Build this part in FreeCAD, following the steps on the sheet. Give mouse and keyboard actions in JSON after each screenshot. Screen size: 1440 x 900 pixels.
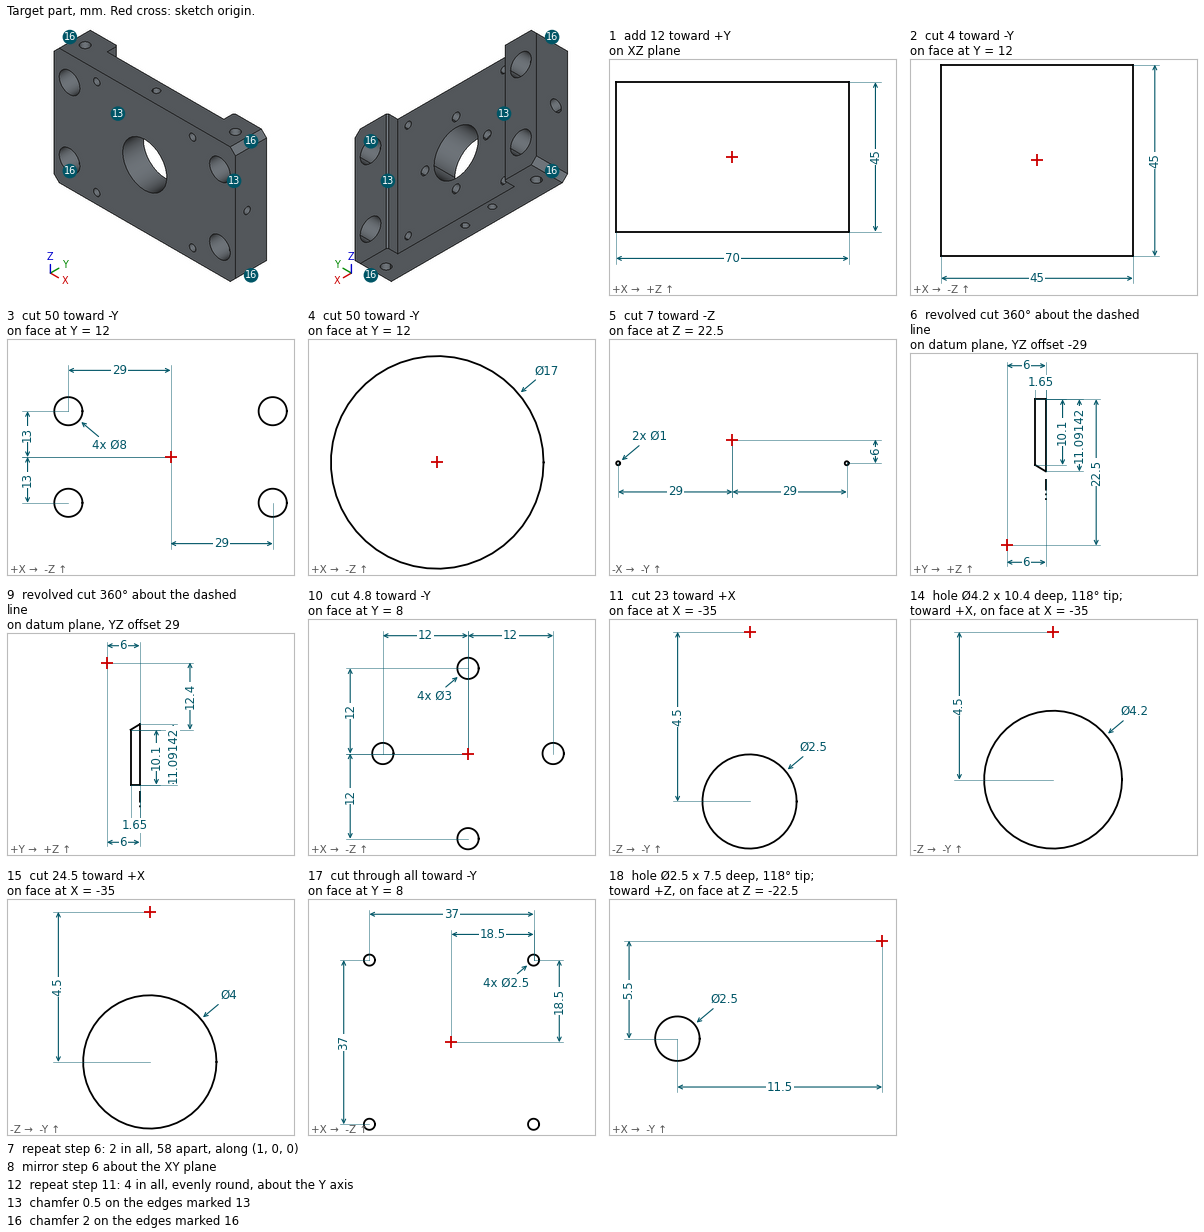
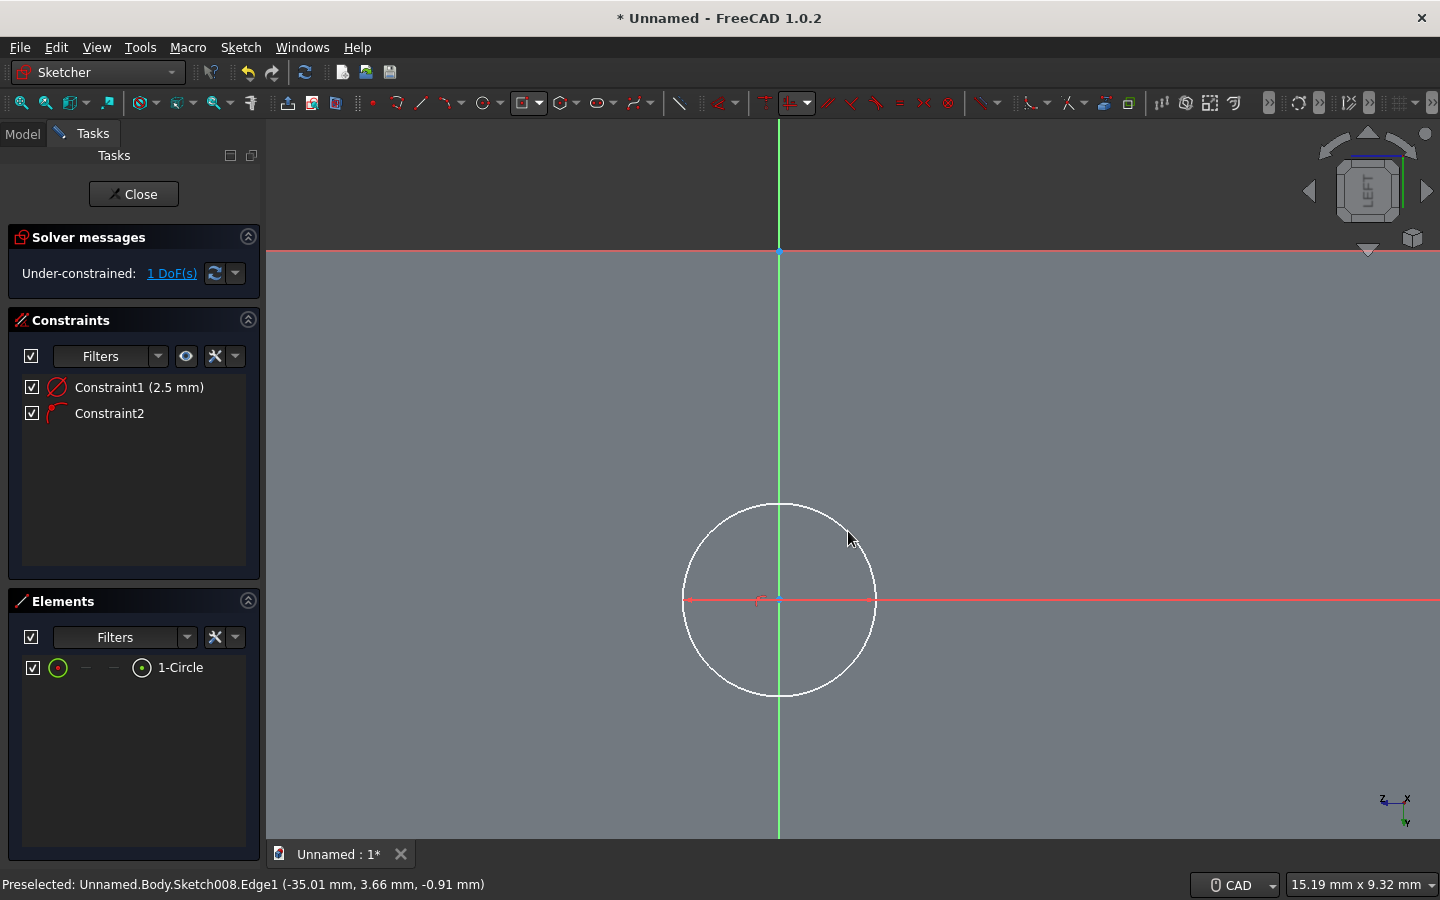
{"action": "left_click", "coordinate": [718, 104]}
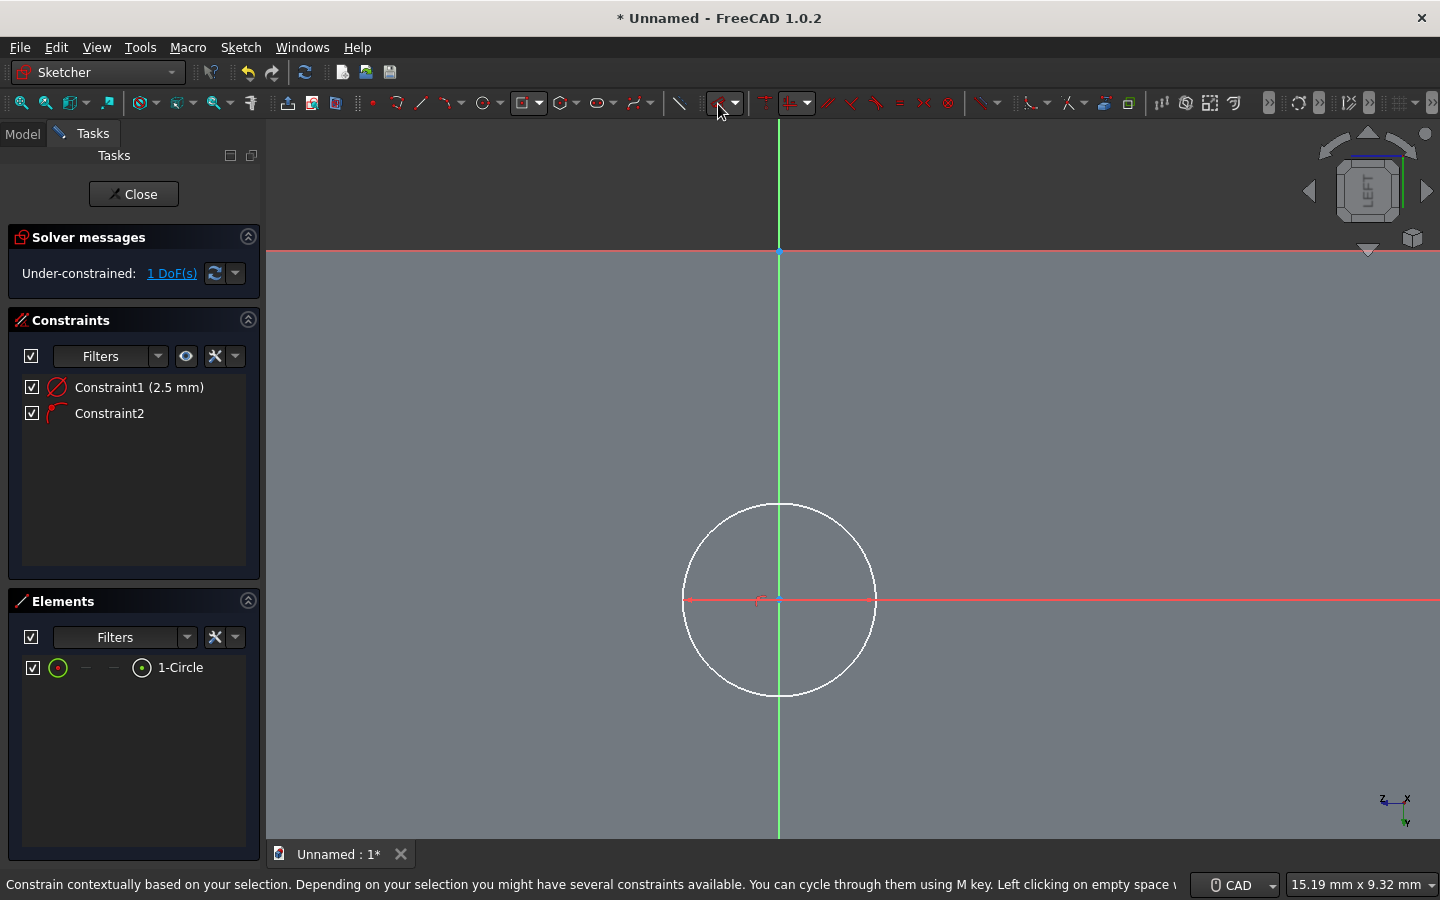
{"action": "left_click", "coordinate": [779, 600]}
{"action": "left_click", "coordinate": [813, 426]}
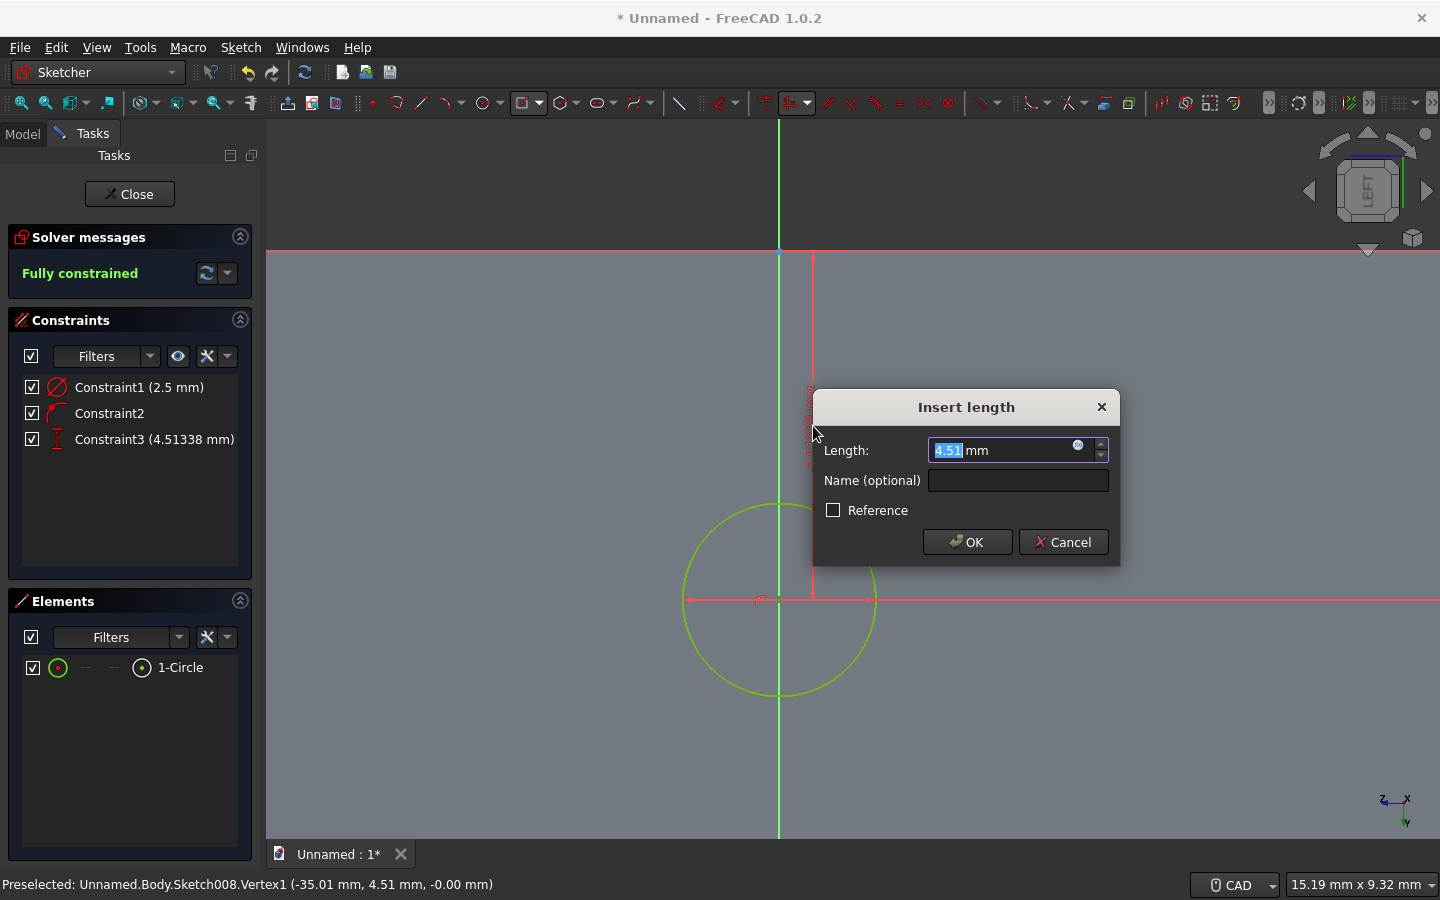
{"action": "type", "text": "4.5"}
{"action": "key", "text": "Return"}
{"action": "key", "text": "Escape"}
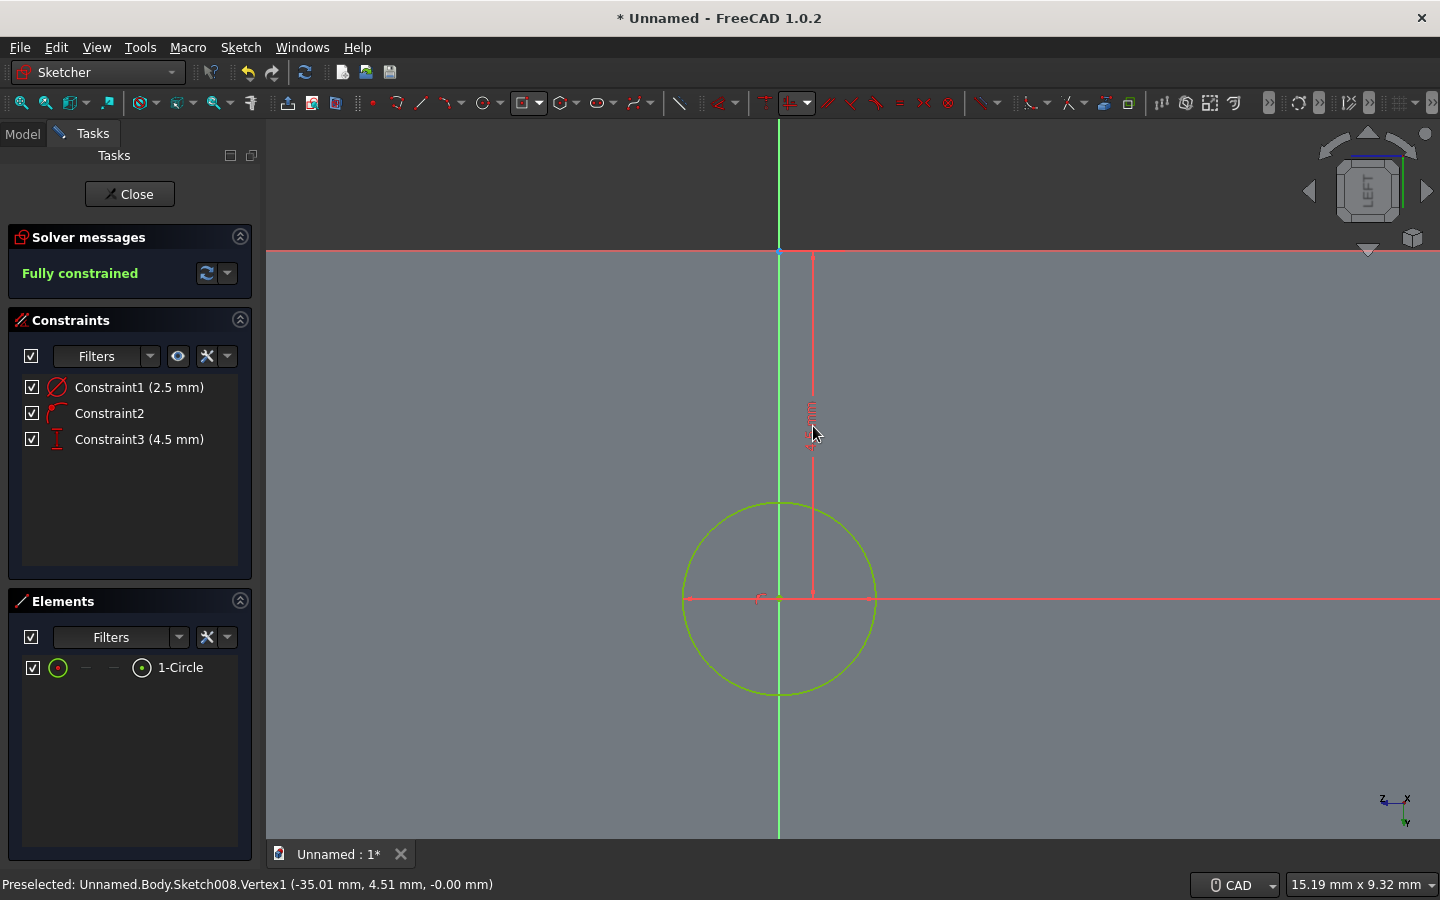
{"action": "left_click", "coordinate": [130, 194]}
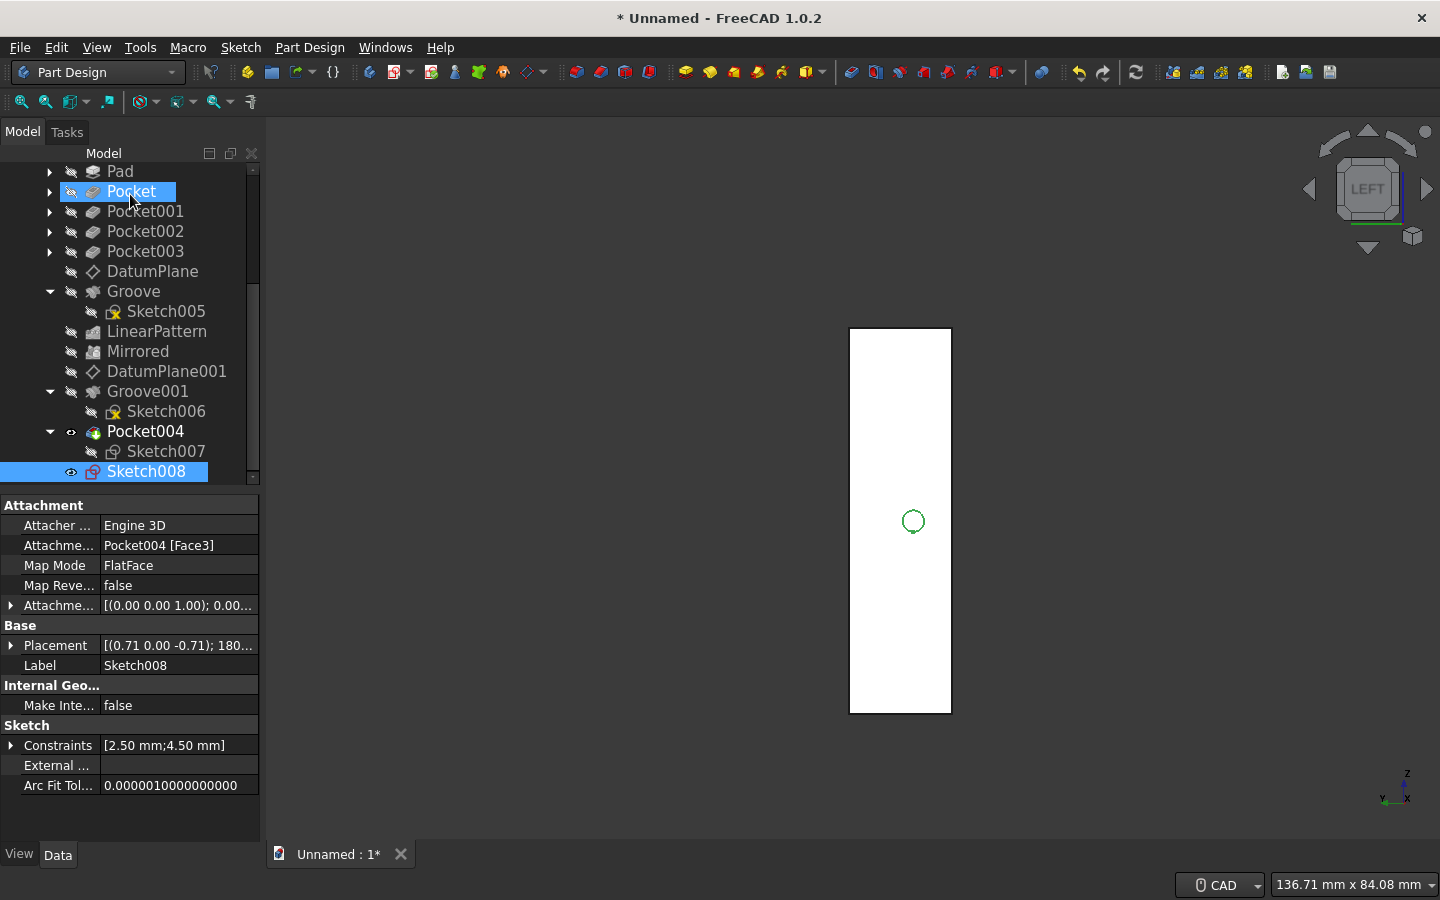
{"action": "left_click", "coordinate": [852, 72]}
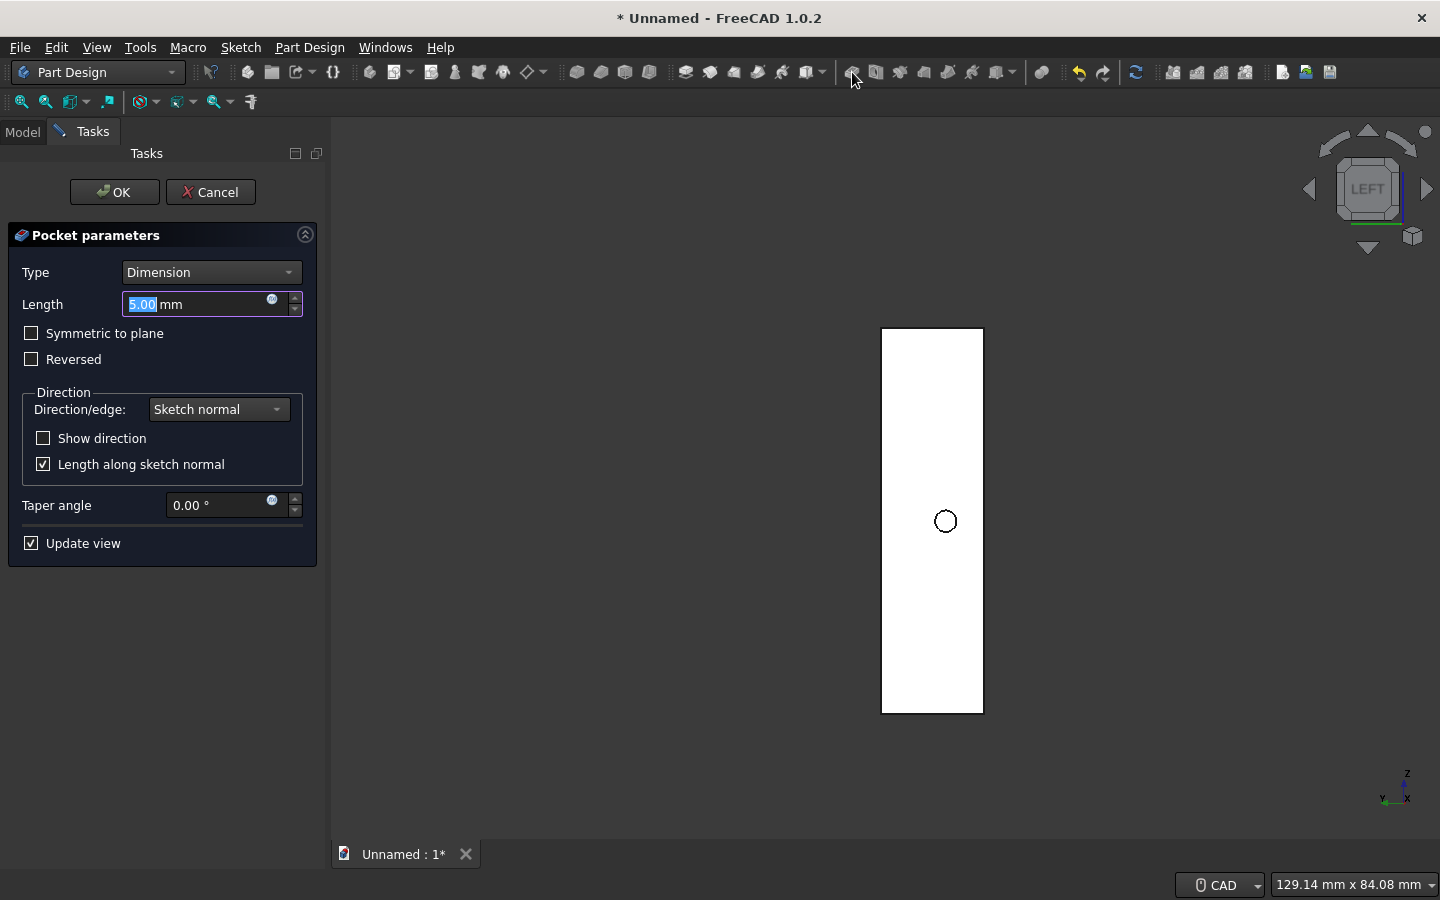
{"action": "type", "text": "23"}
{"action": "key", "text": "Tab"}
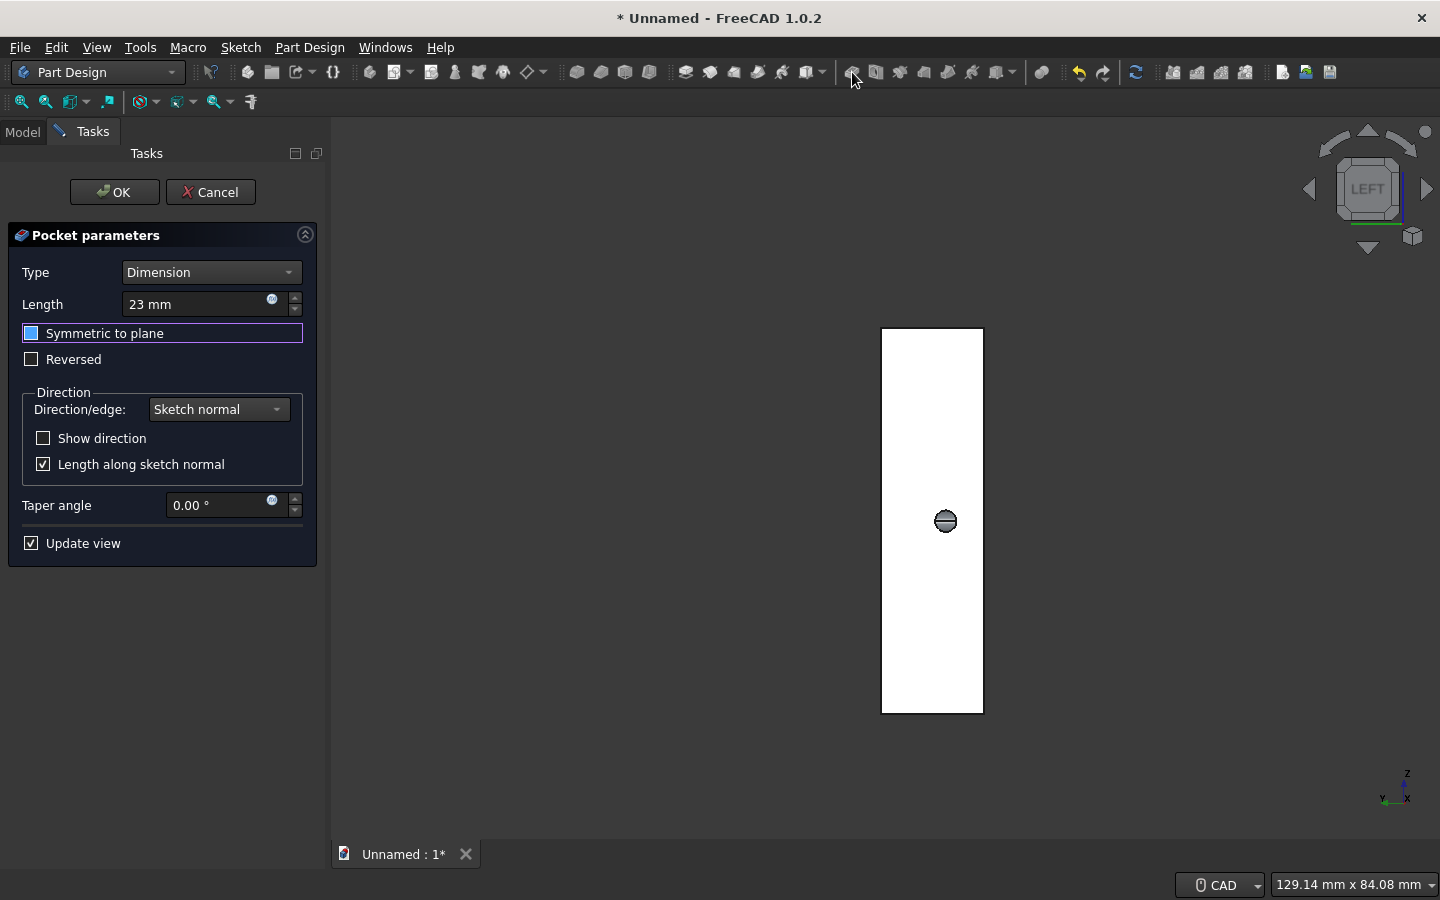
{"action": "left_click", "coordinate": [115, 192]}